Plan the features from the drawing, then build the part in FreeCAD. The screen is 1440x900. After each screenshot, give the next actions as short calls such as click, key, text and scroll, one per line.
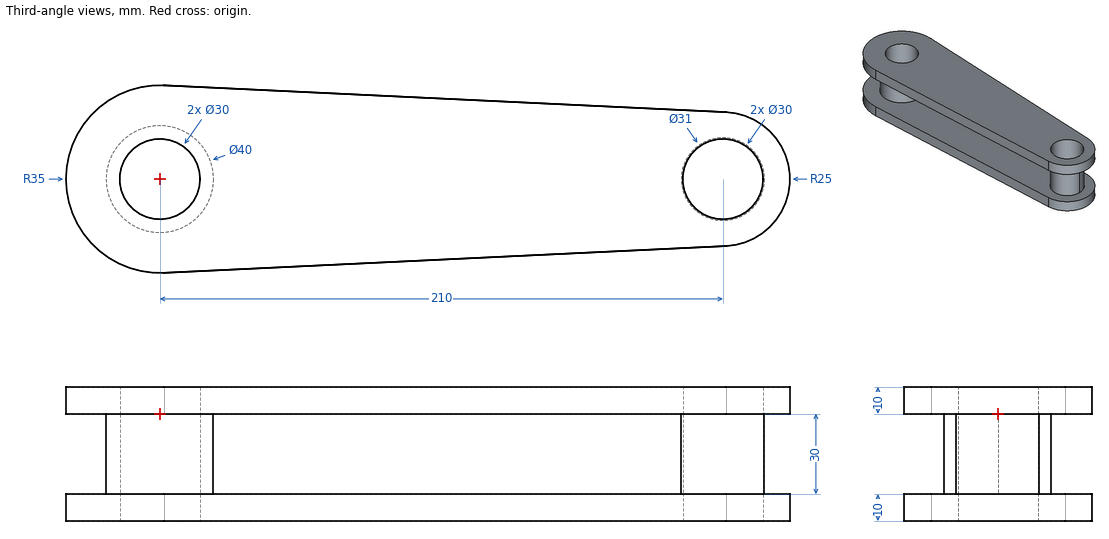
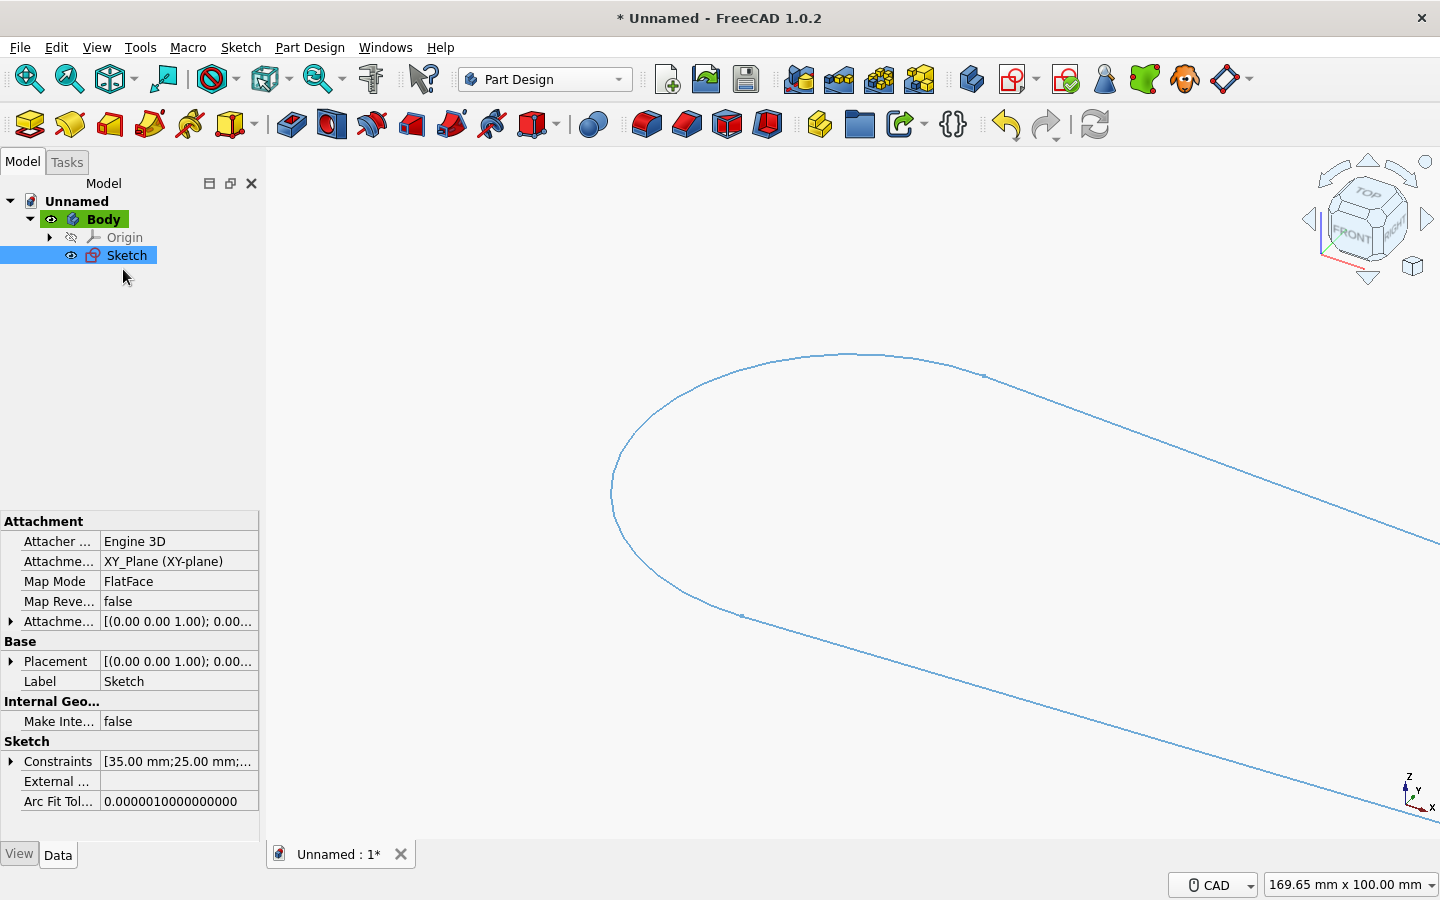
click(30, 124)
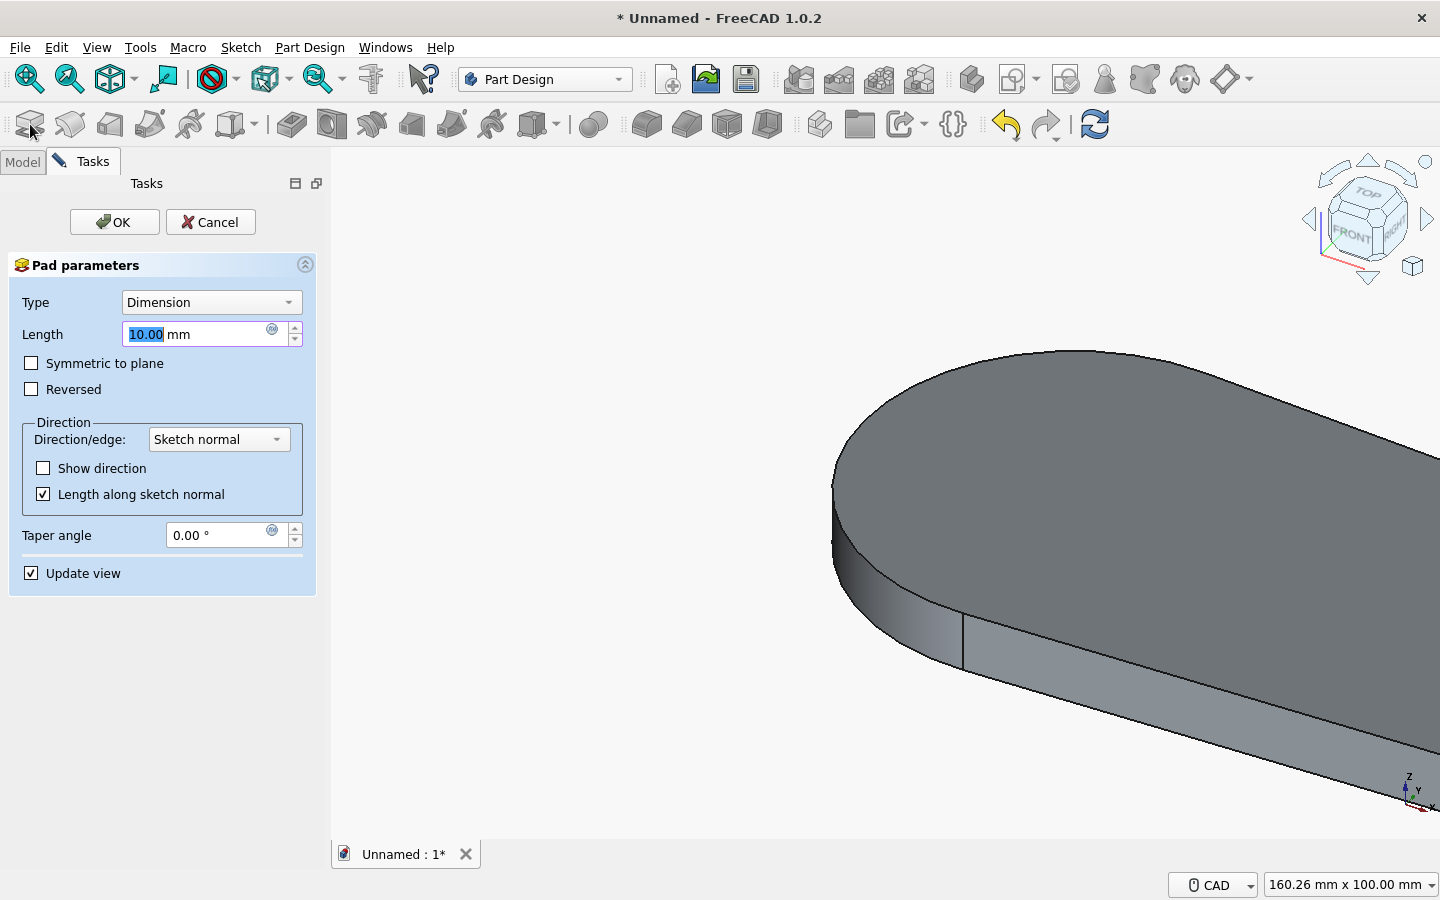
text(10)
key(Tab)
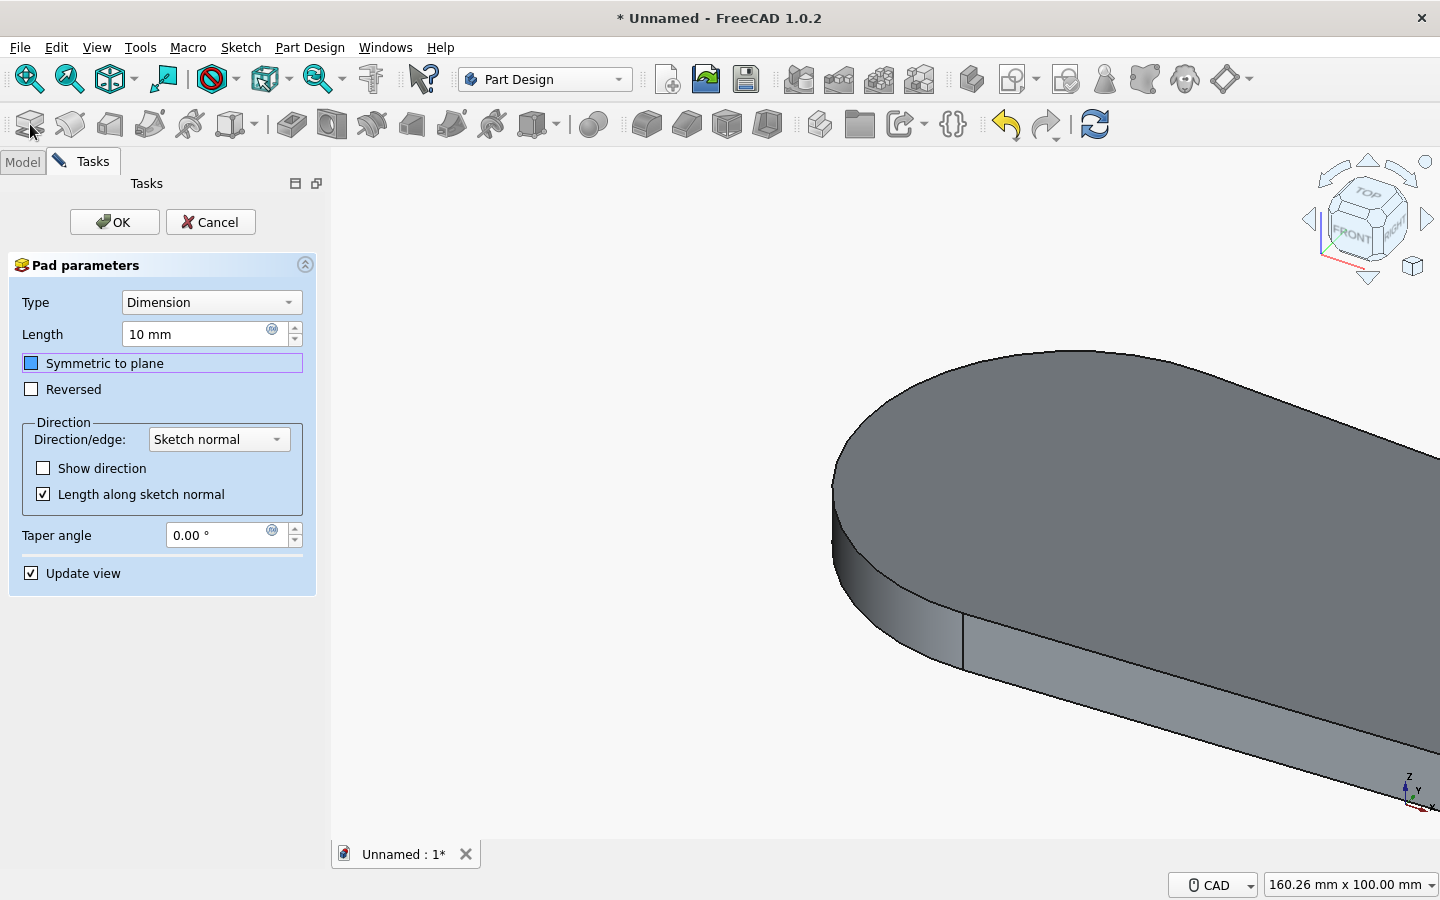
click(115, 222)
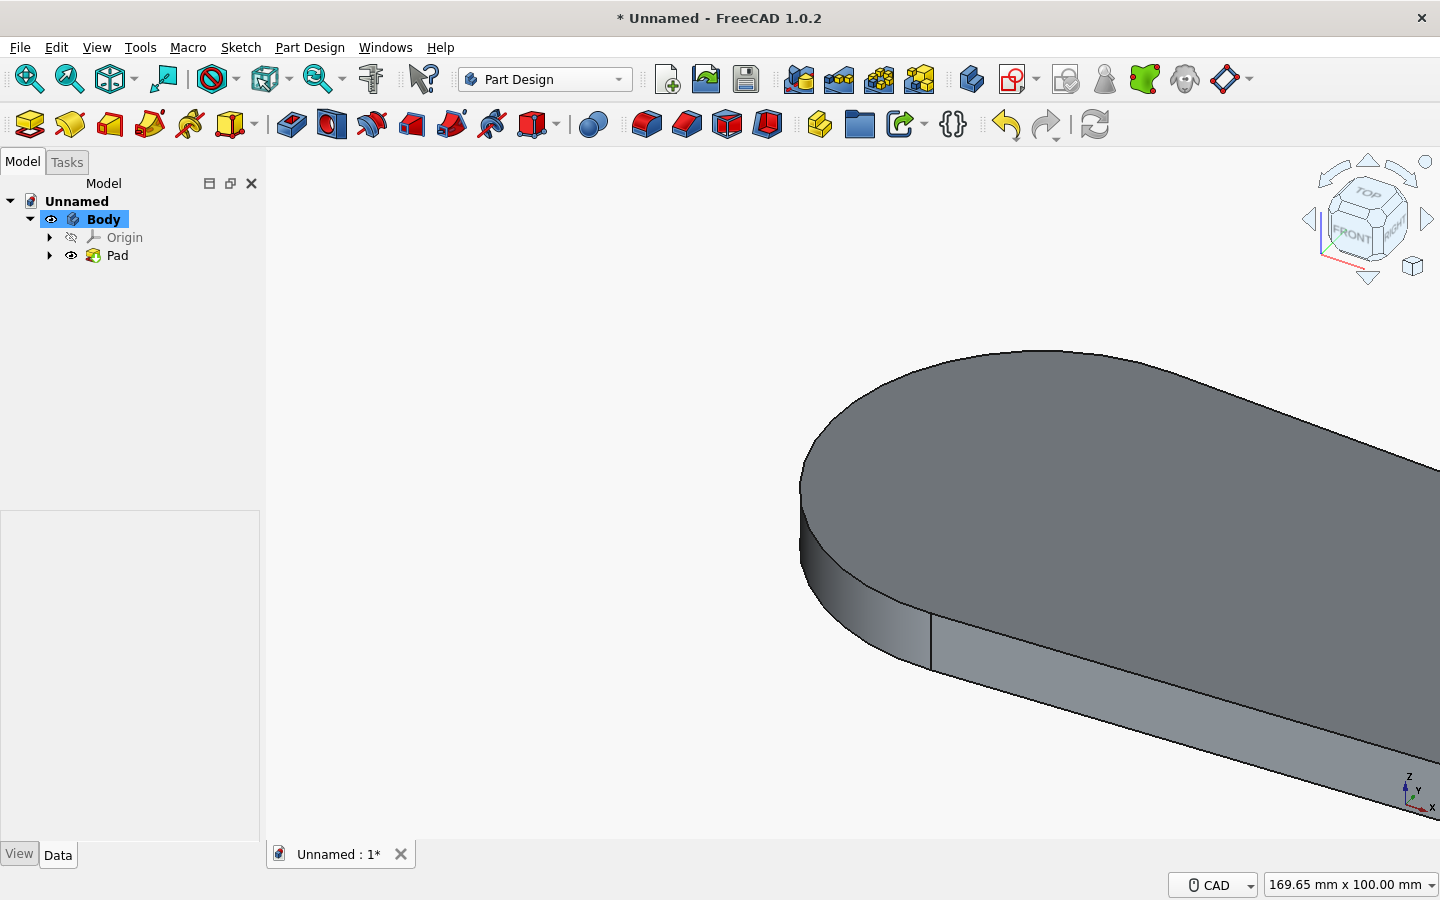
click(30, 80)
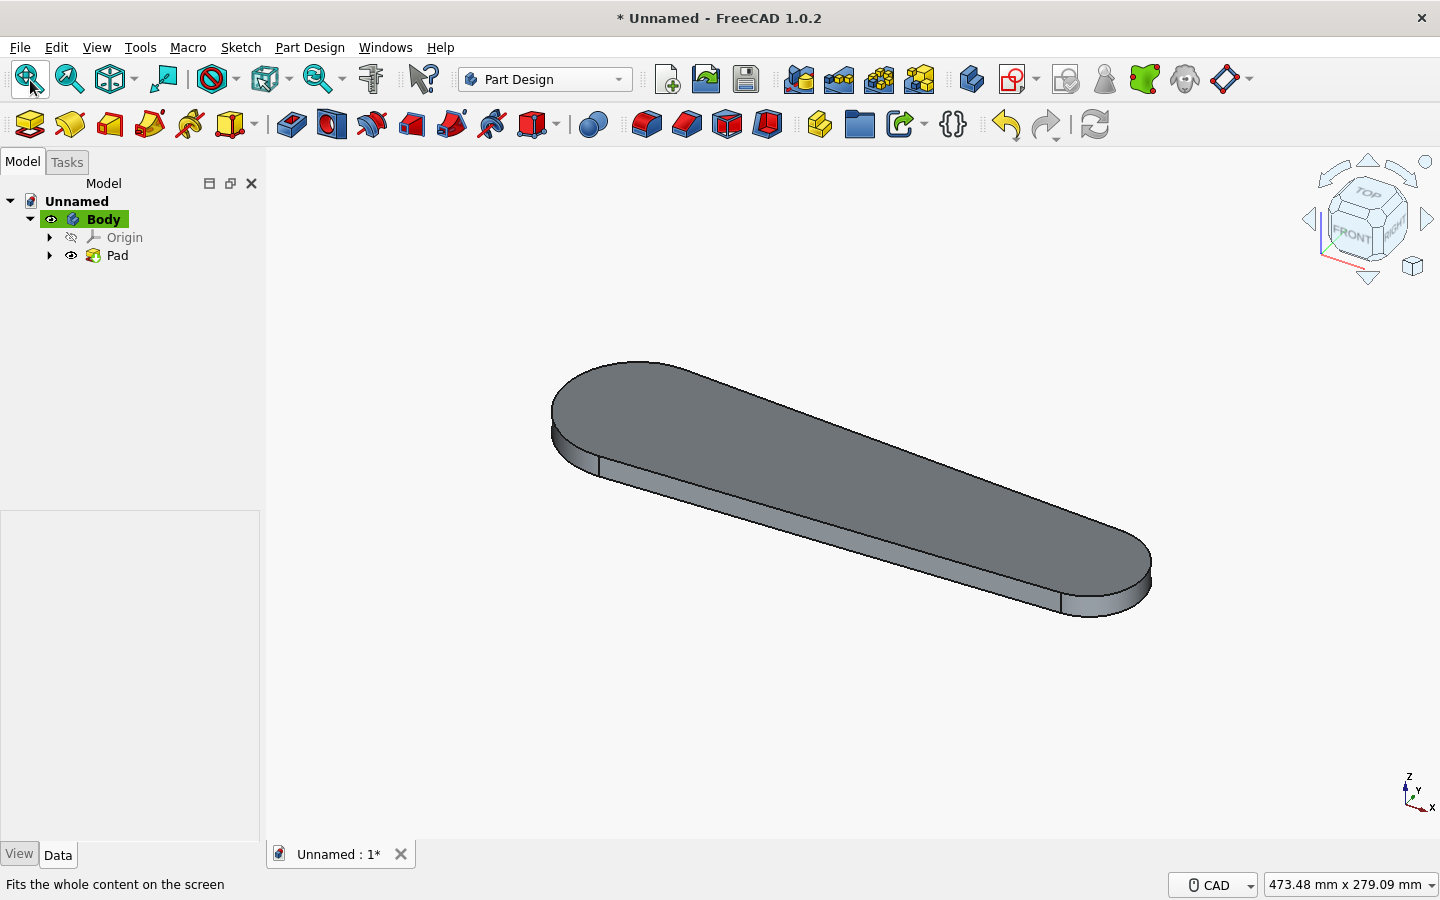
key(5)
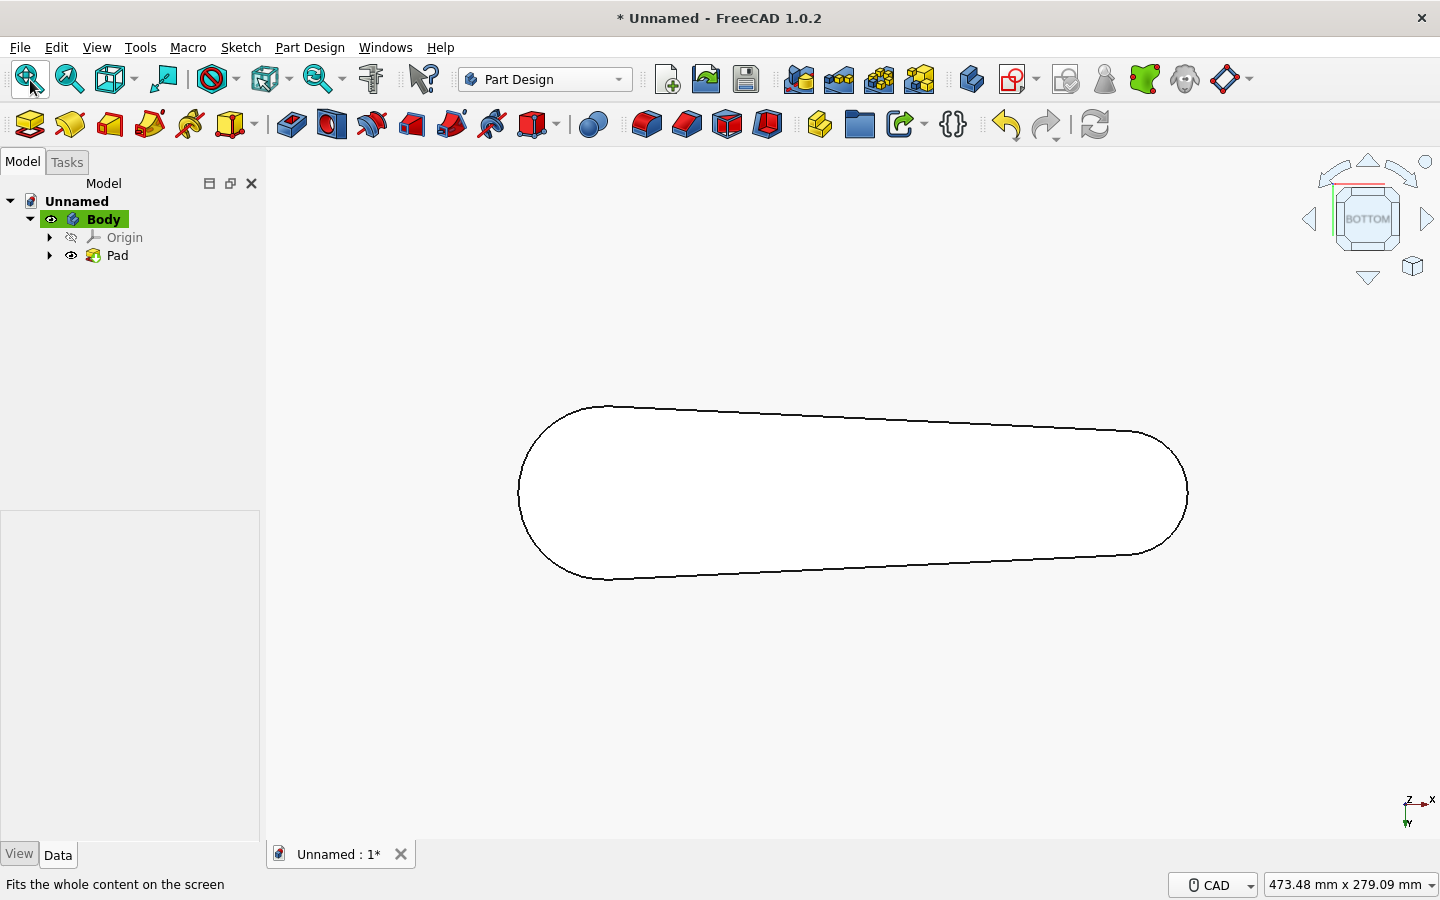
click(662, 492)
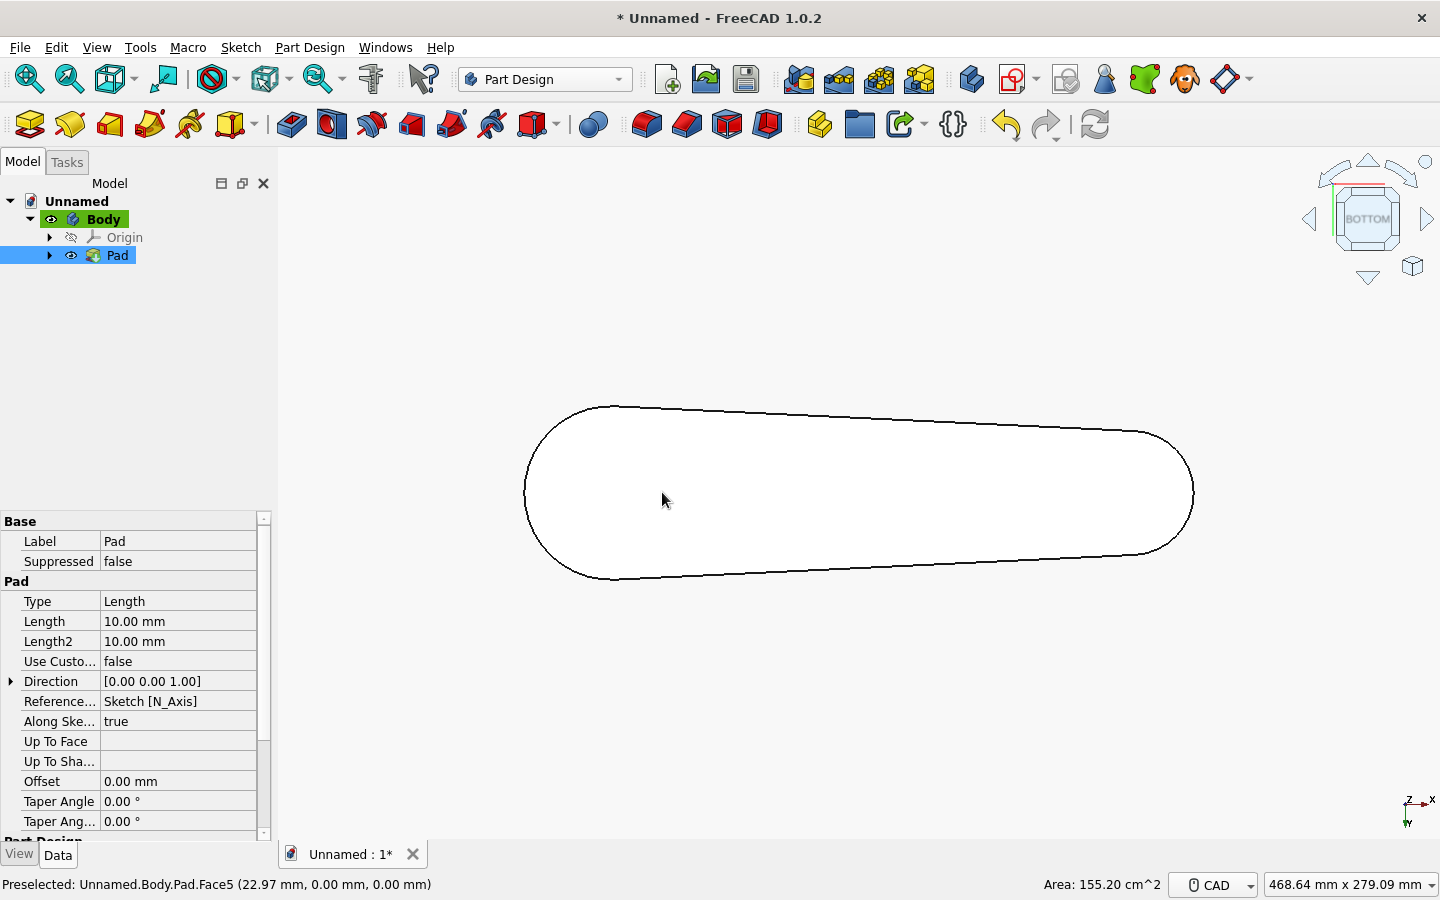
click(1012, 80)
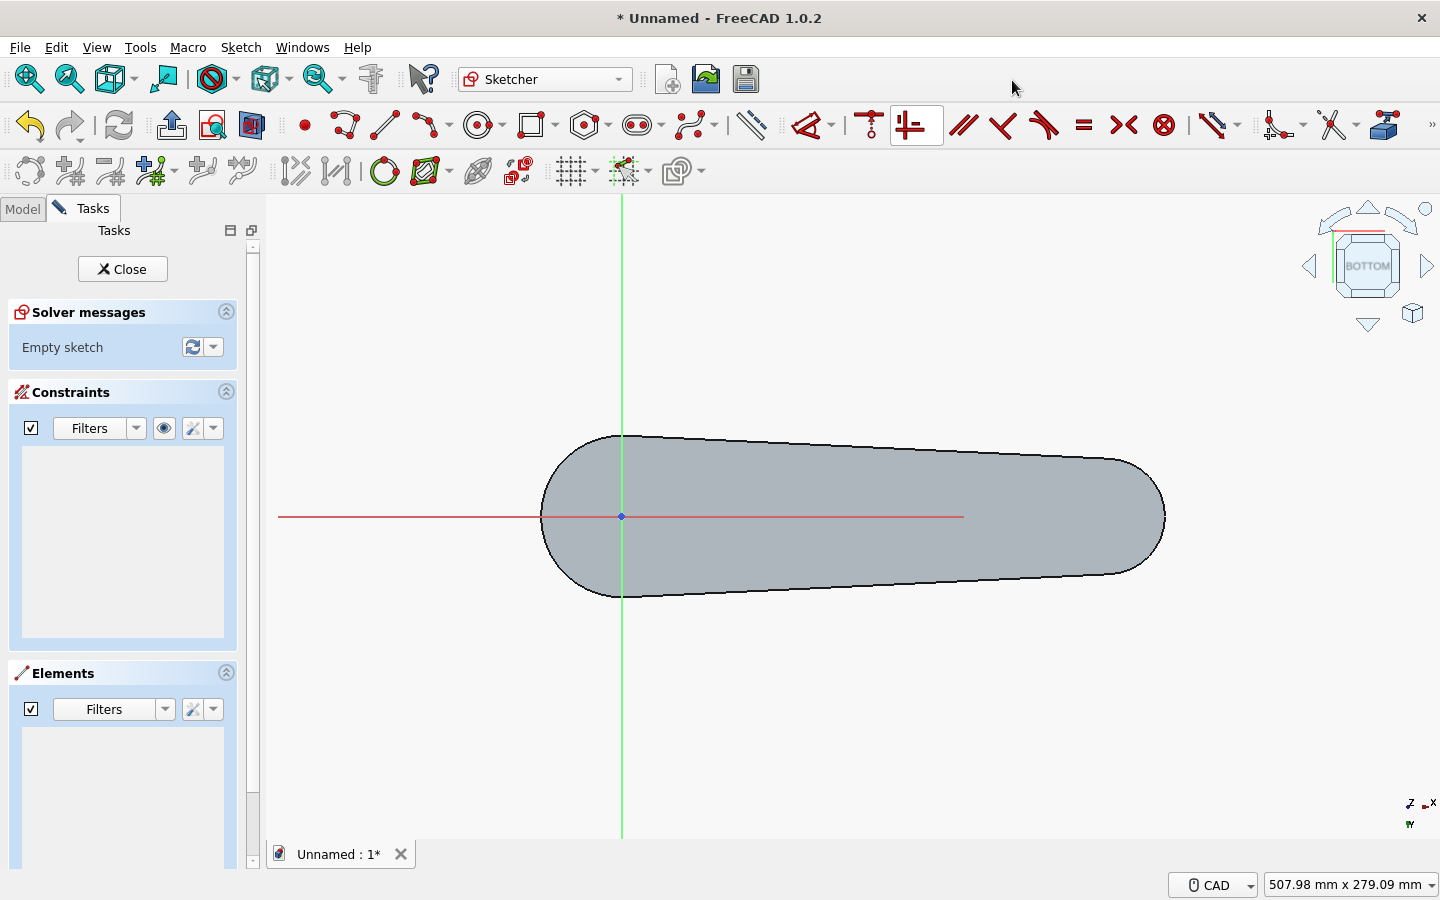
click(478, 126)